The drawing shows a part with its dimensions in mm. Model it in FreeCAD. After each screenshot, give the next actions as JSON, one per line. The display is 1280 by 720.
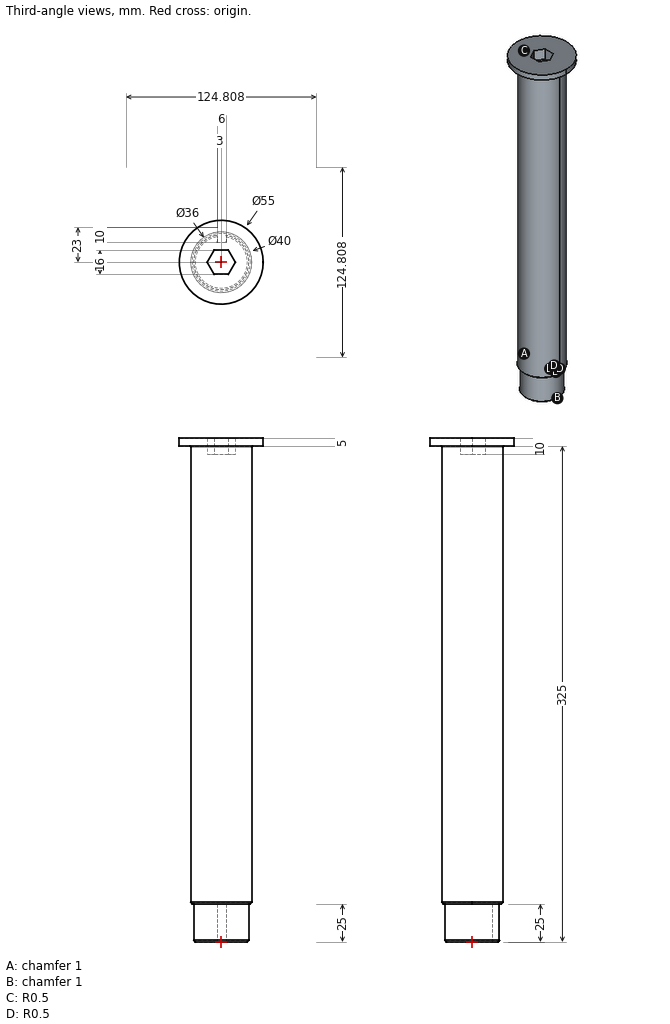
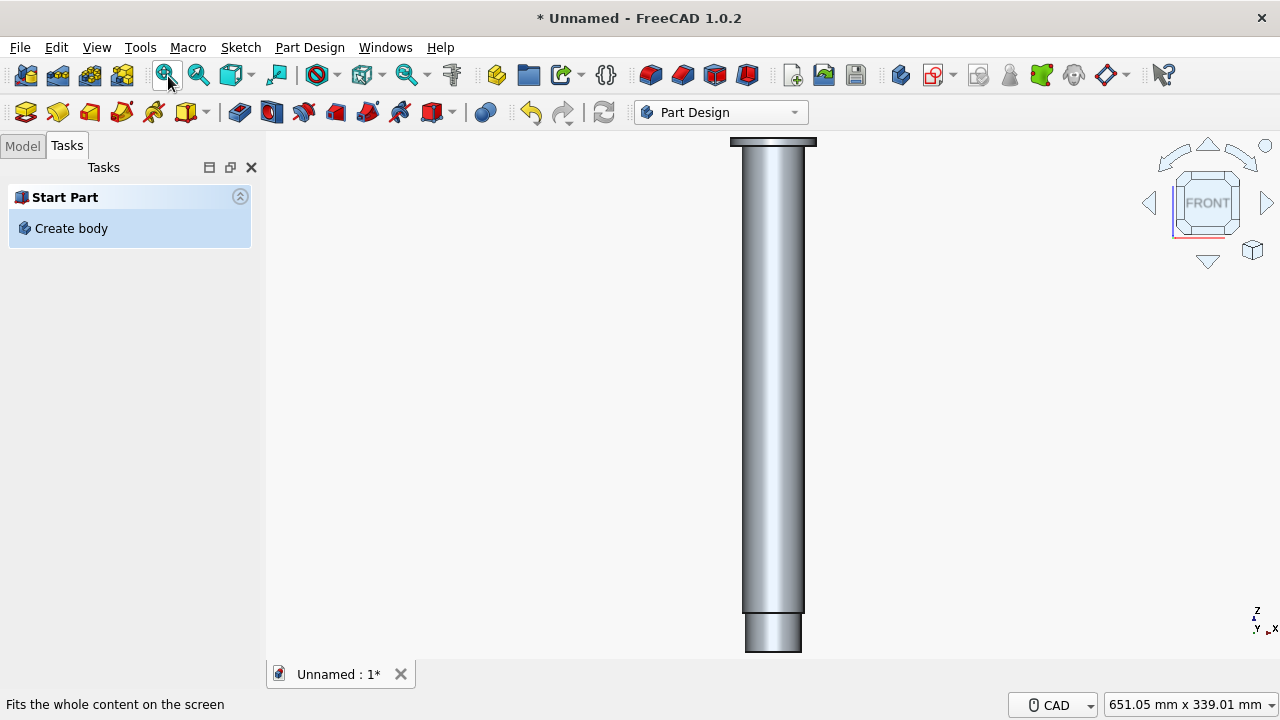
{"action": "left_click", "coordinate": [742, 612]}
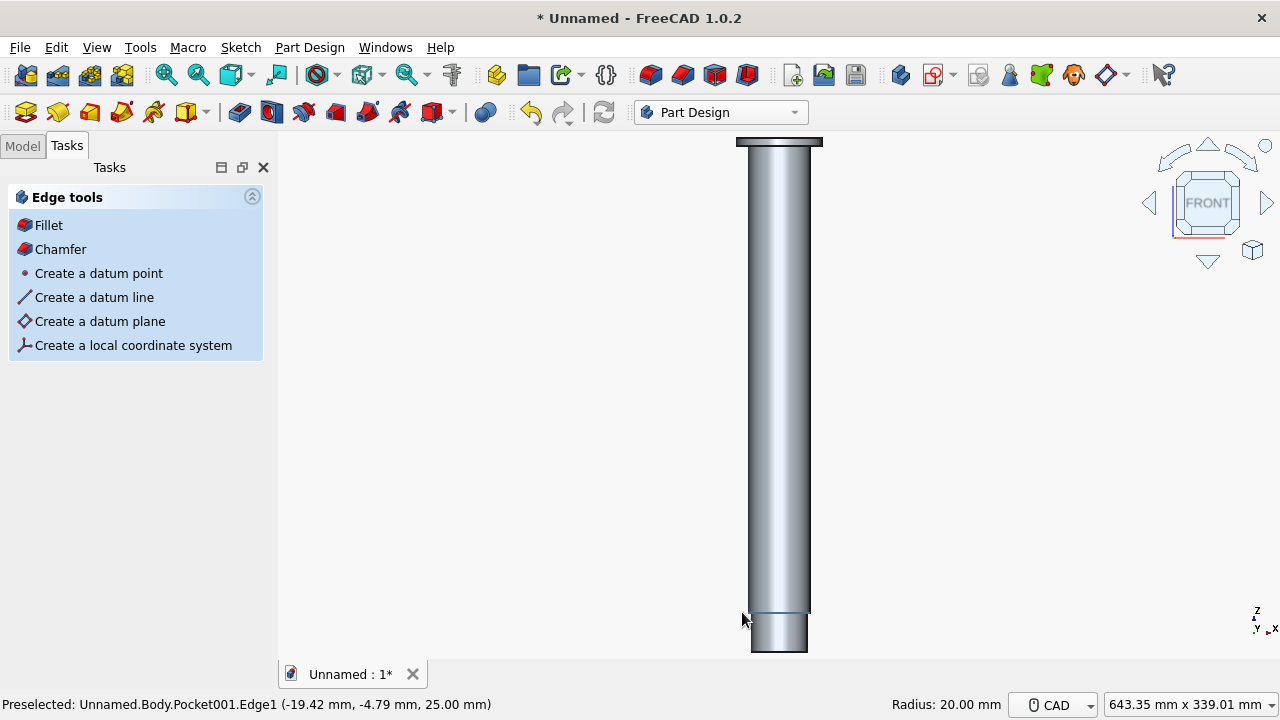
{"action": "left_click", "coordinate": [684, 76]}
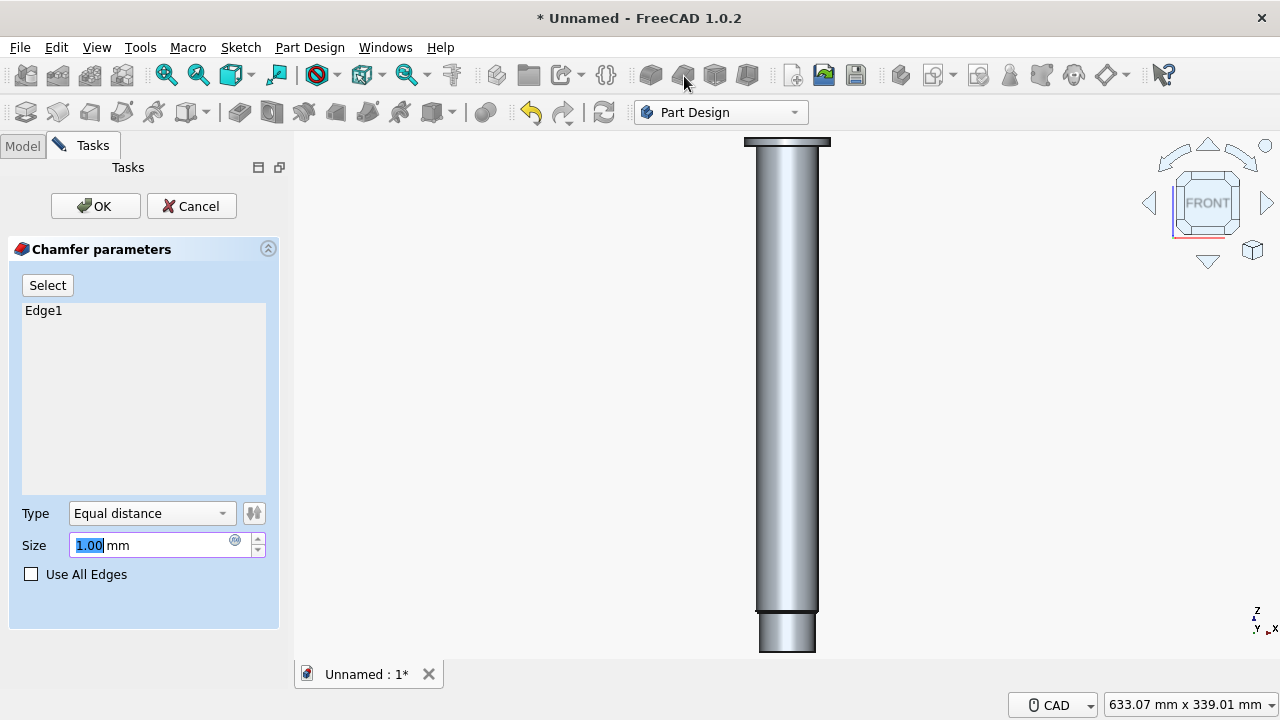
{"action": "type", "text": "1"}
{"action": "key", "text": "Tab"}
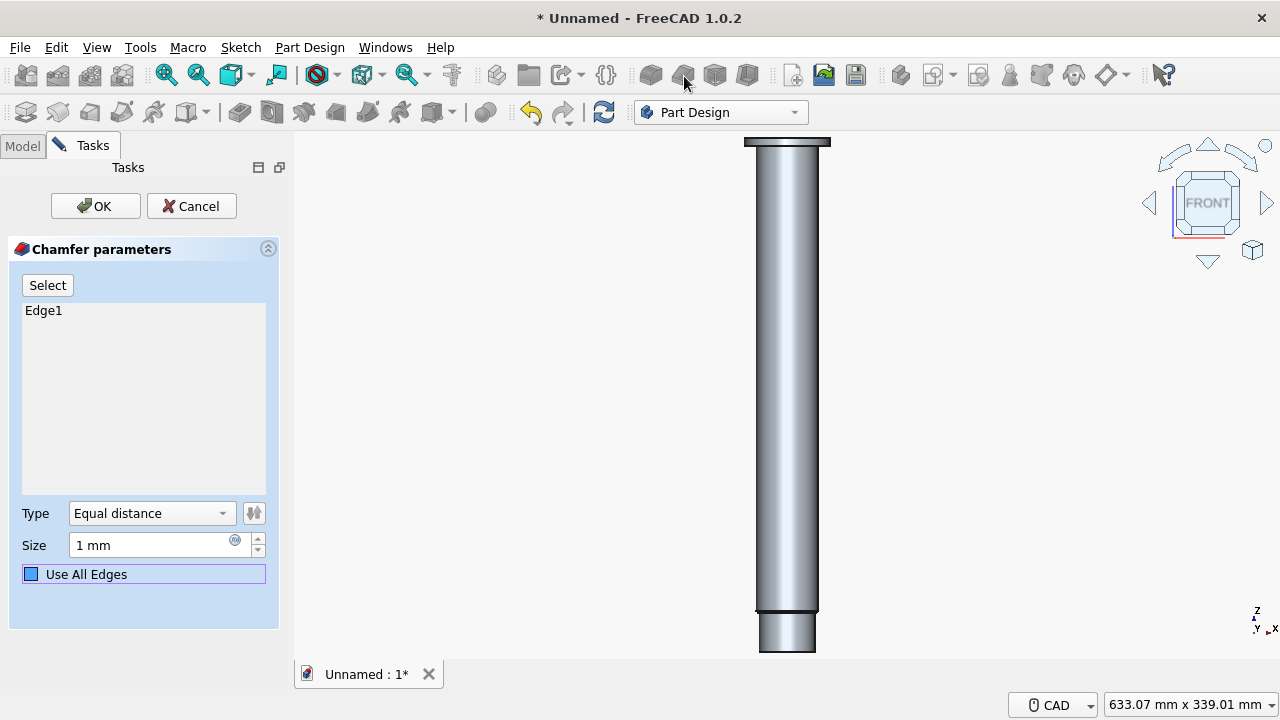
{"action": "left_click", "coordinate": [96, 206]}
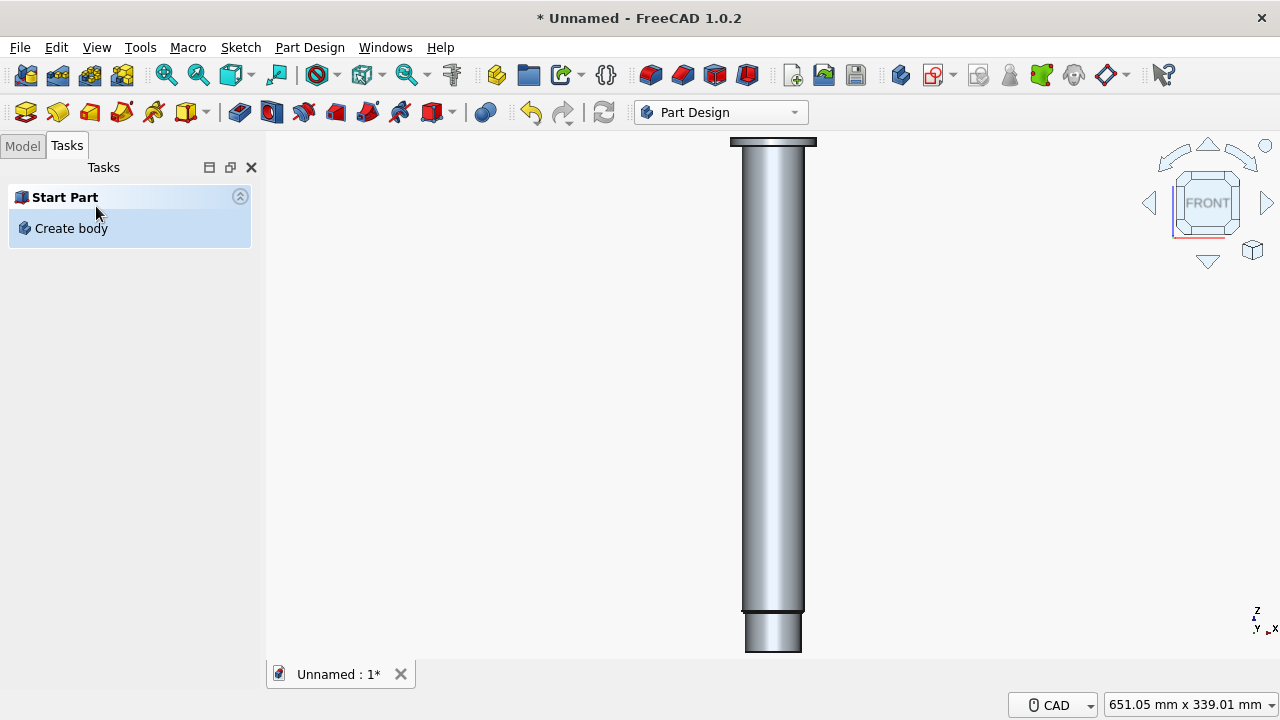
{"action": "key", "text": "0"}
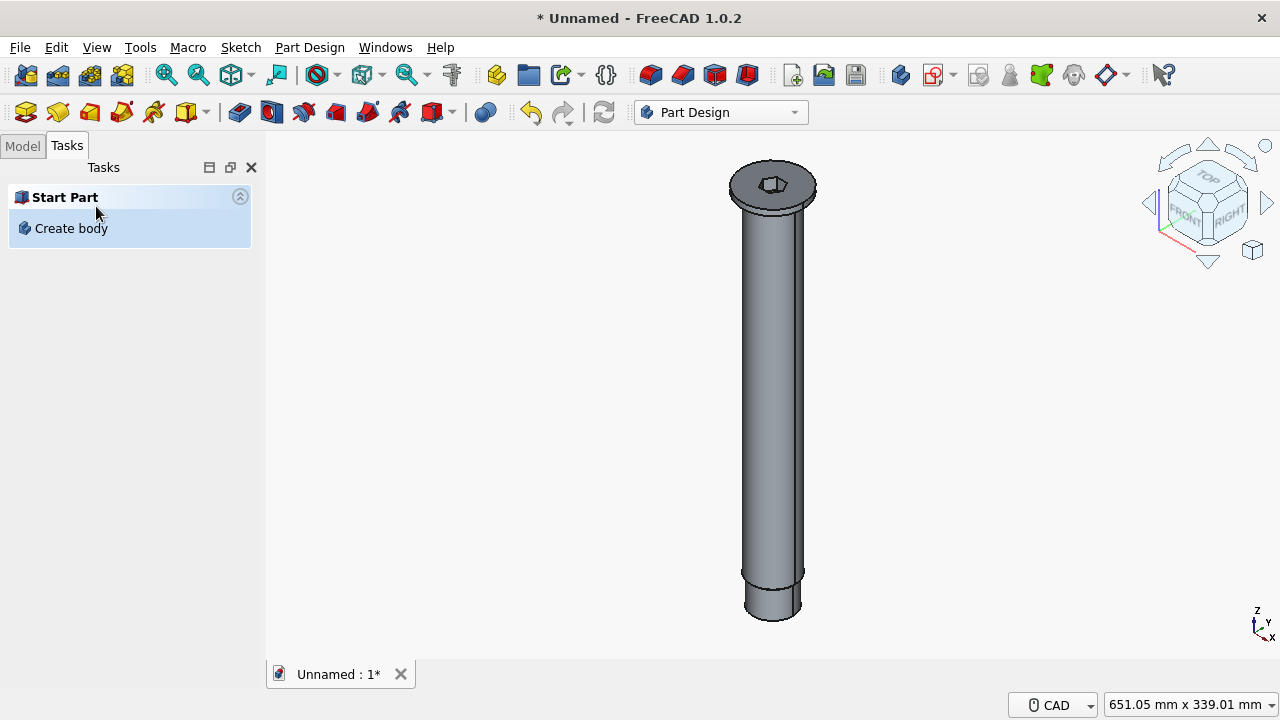
{"action": "left_click", "coordinate": [748, 611]}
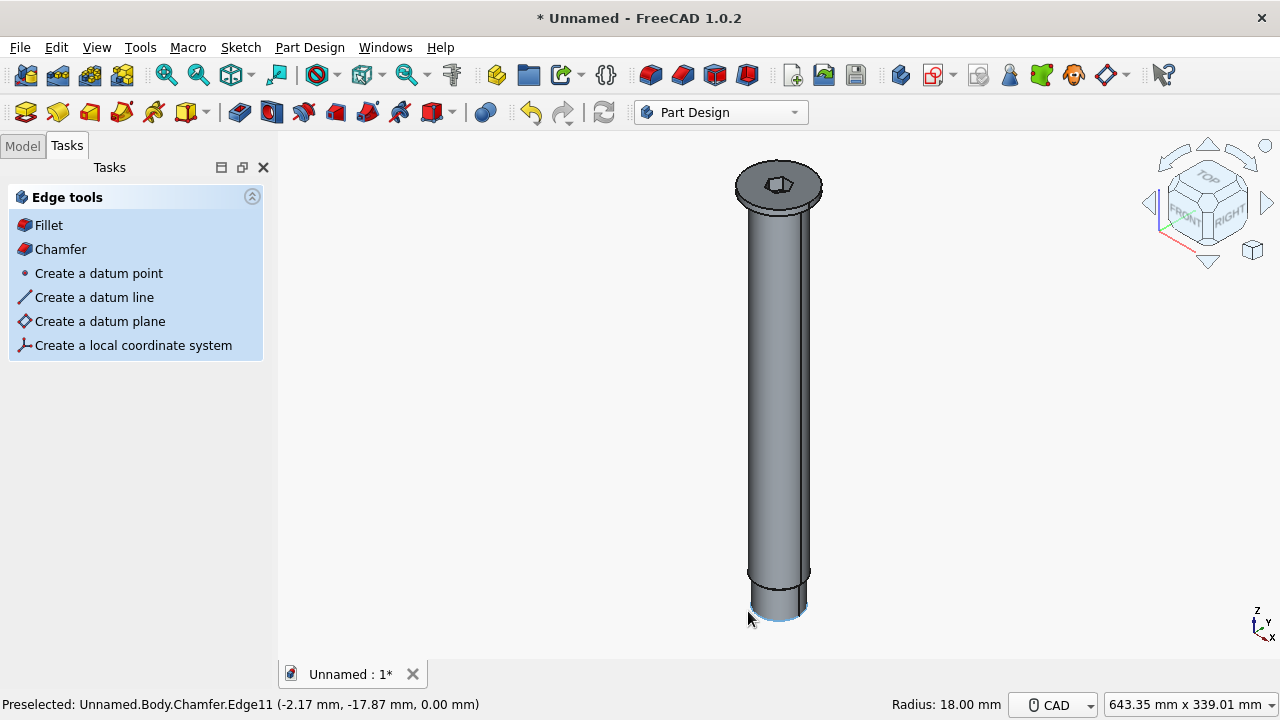
{"action": "left_click", "coordinate": [684, 76]}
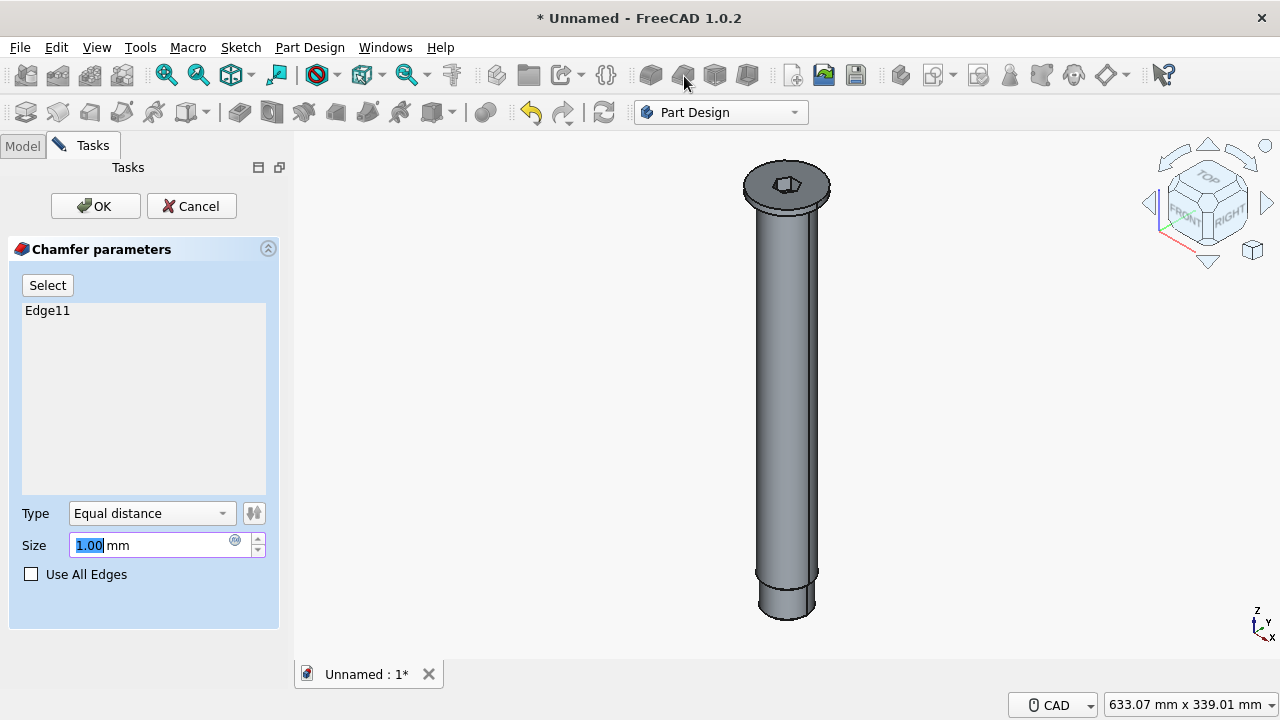
{"action": "type", "text": "1"}
{"action": "key", "text": "Tab"}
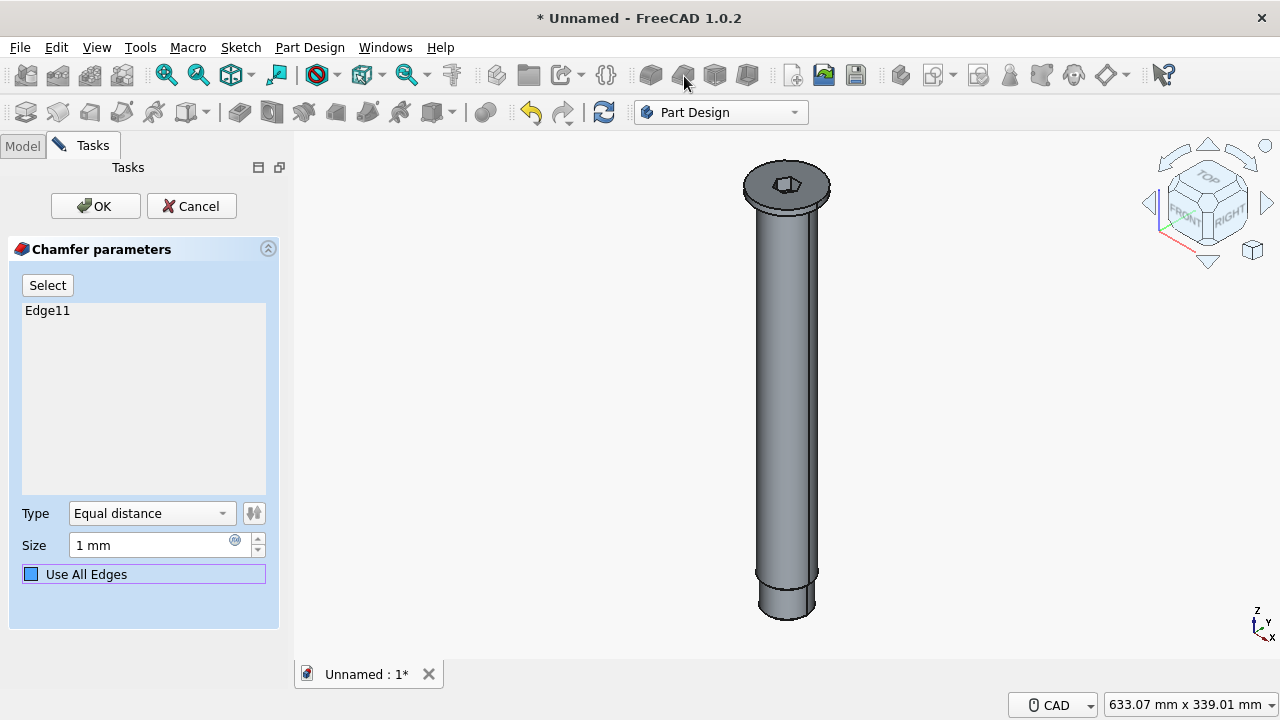
{"action": "left_click", "coordinate": [96, 206]}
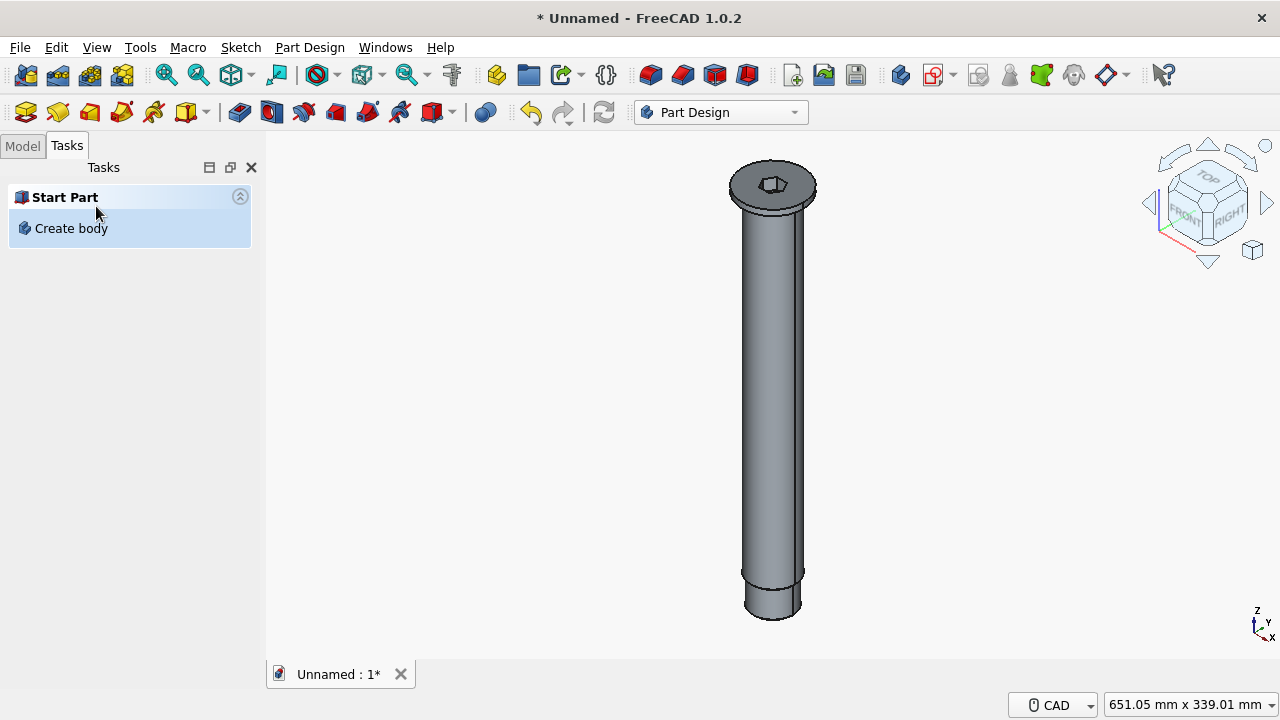
{"action": "key", "text": "2"}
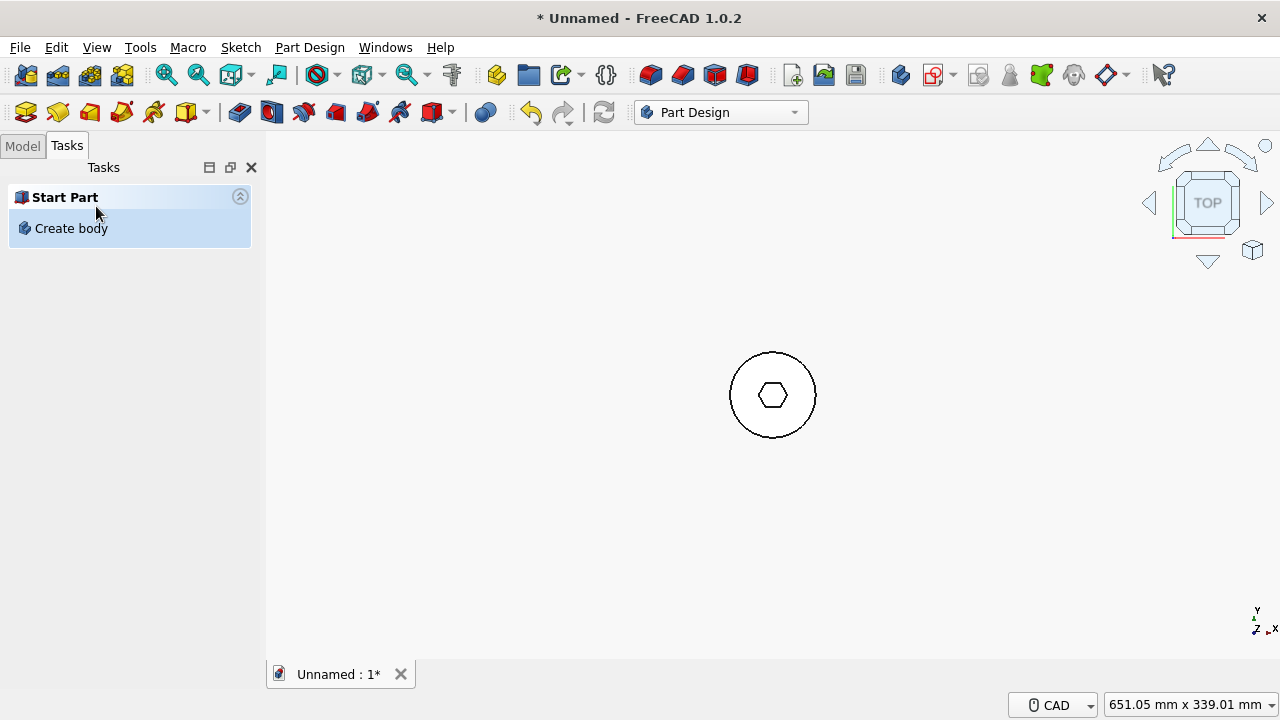
{"action": "left_click", "coordinate": [168, 76]}